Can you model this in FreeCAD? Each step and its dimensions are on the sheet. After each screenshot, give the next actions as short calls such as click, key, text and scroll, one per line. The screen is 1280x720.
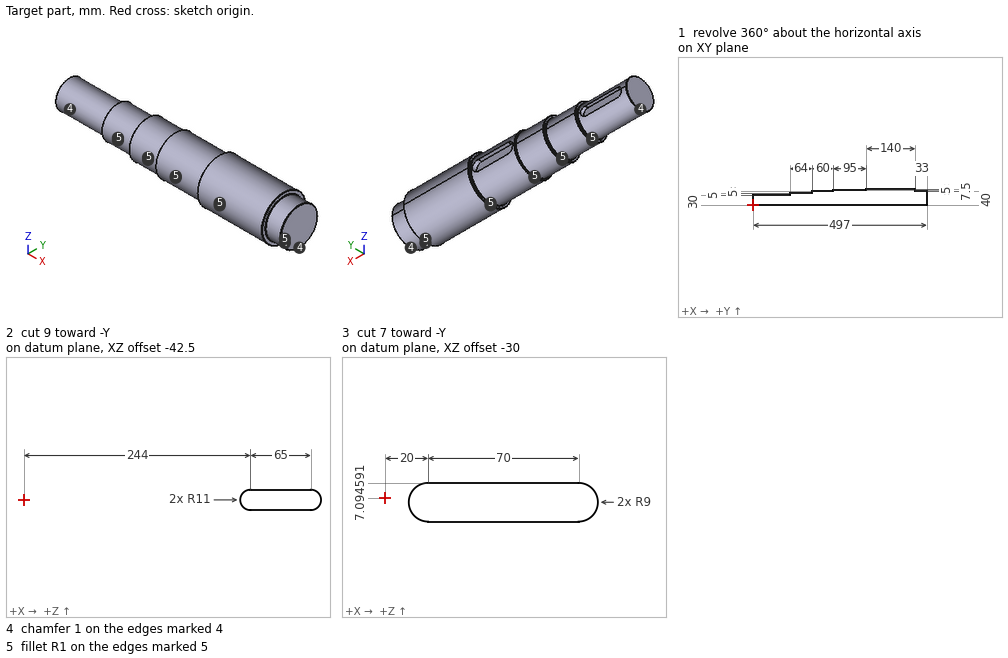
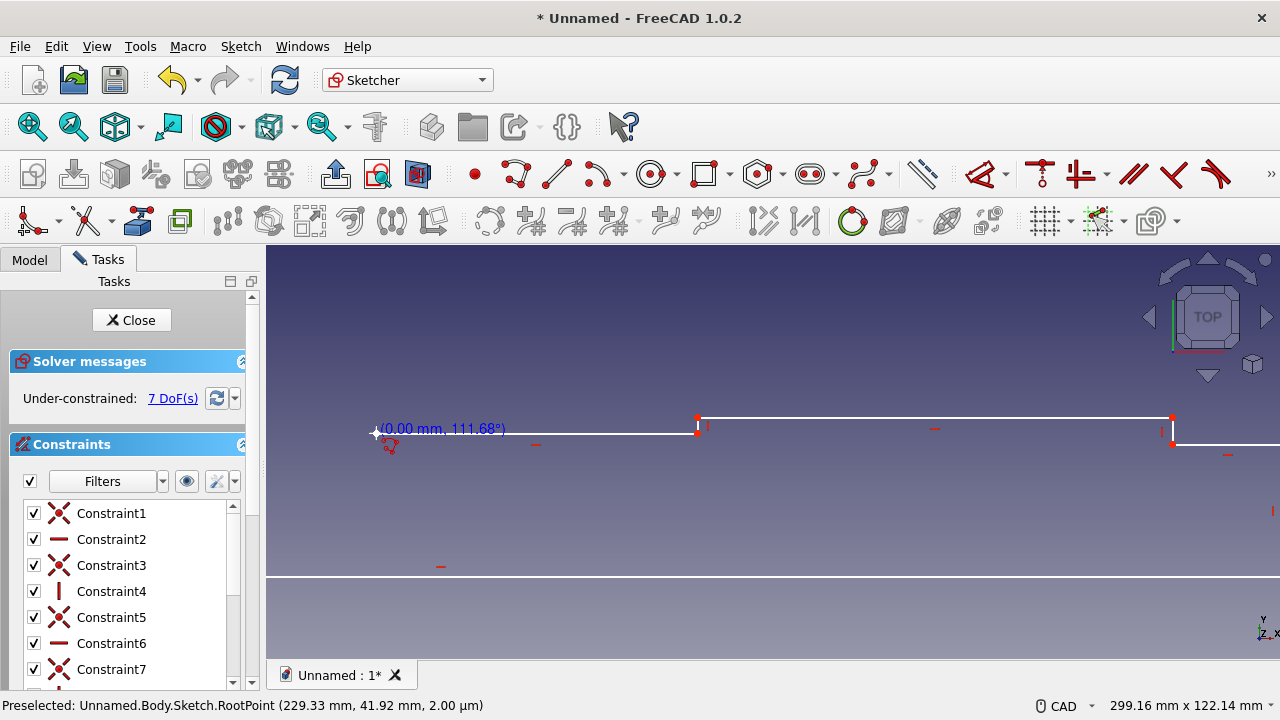
scroll(376, 442, up, 4)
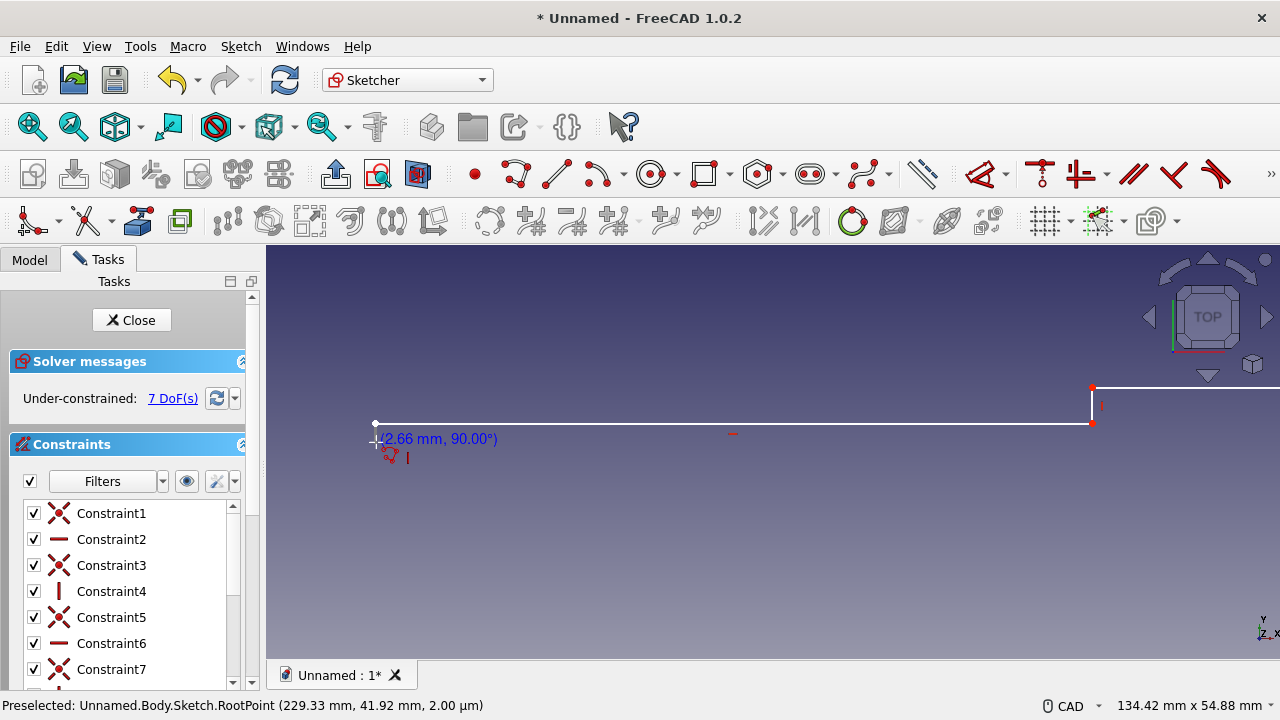
click(376, 440)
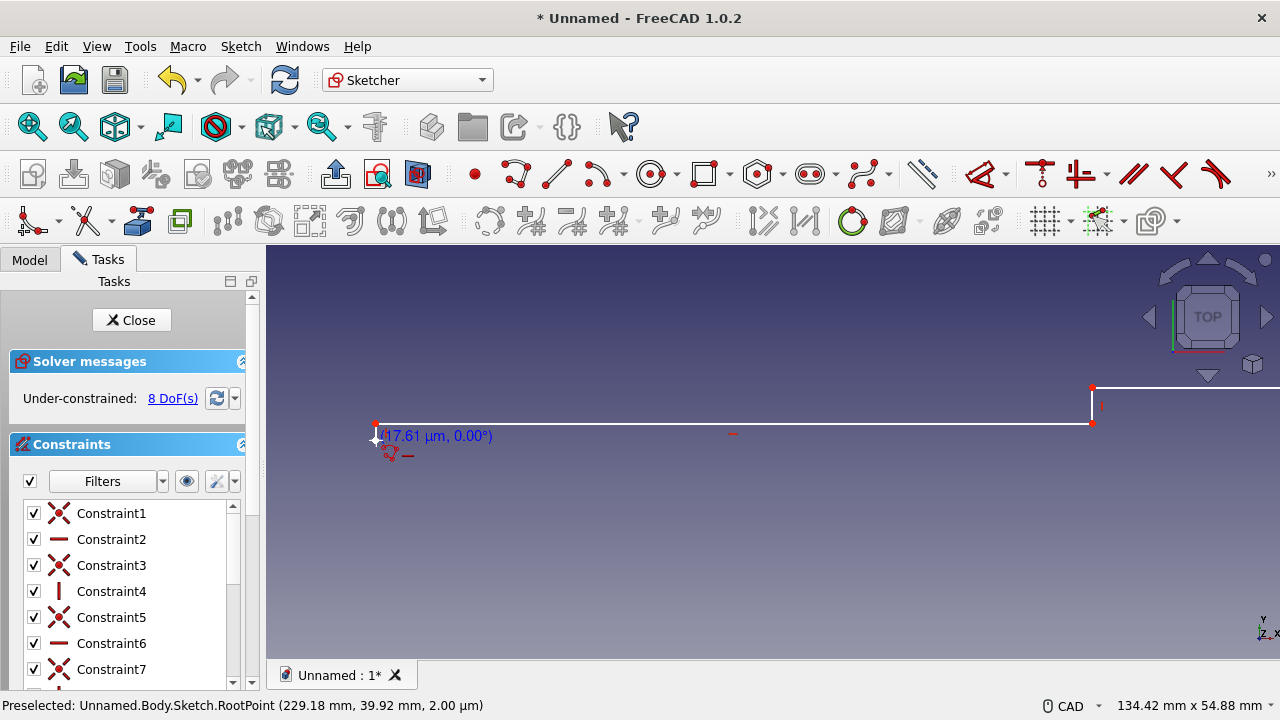
scroll(740, 430, down, 9)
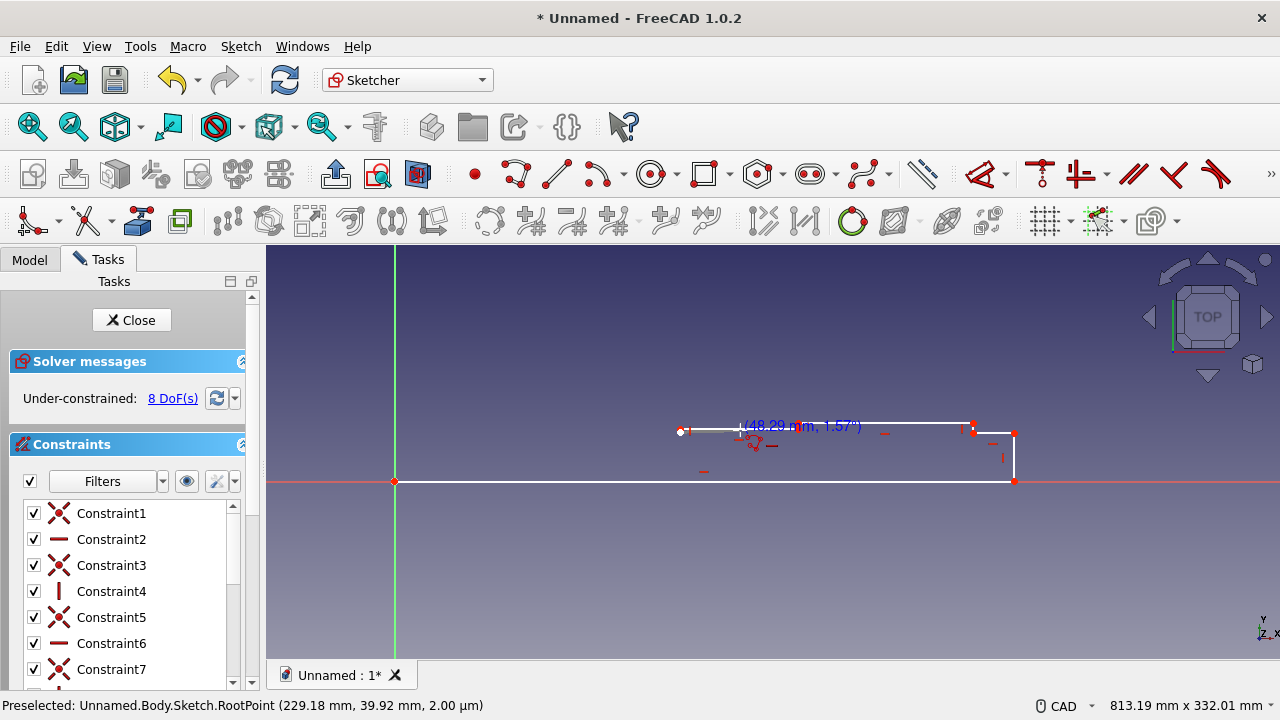
click(605, 432)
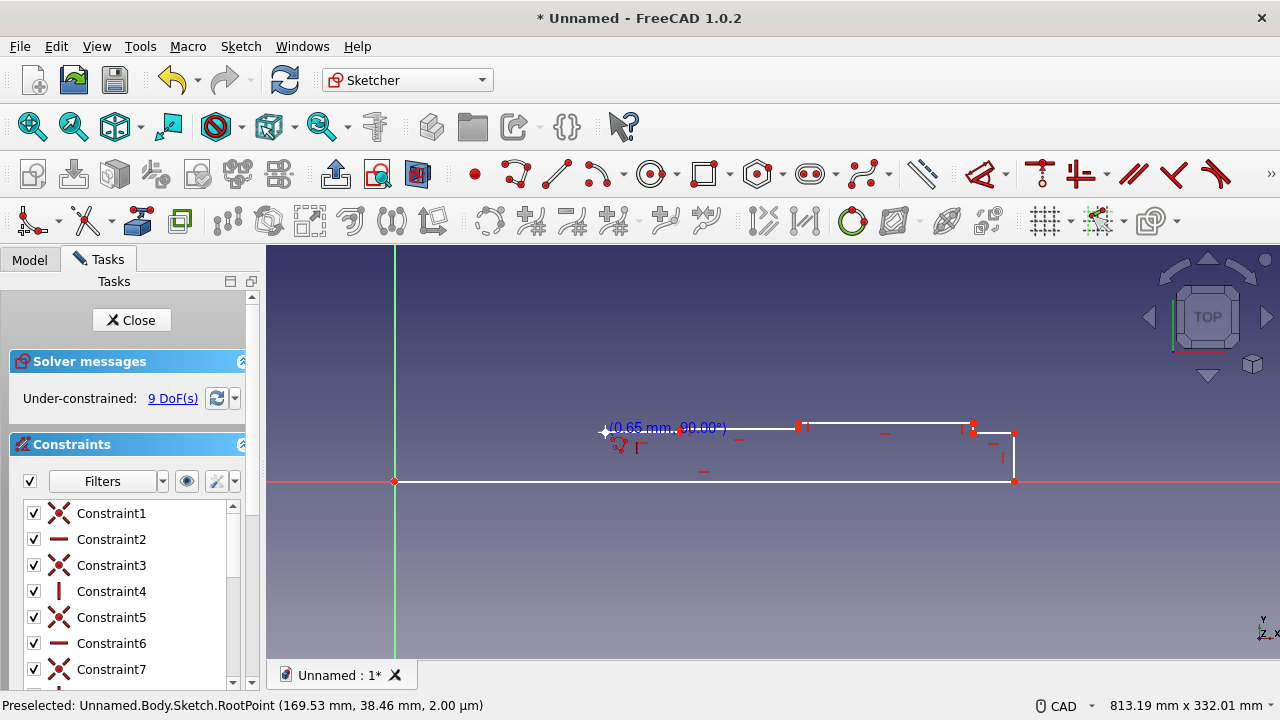
scroll(605, 438, up, 5)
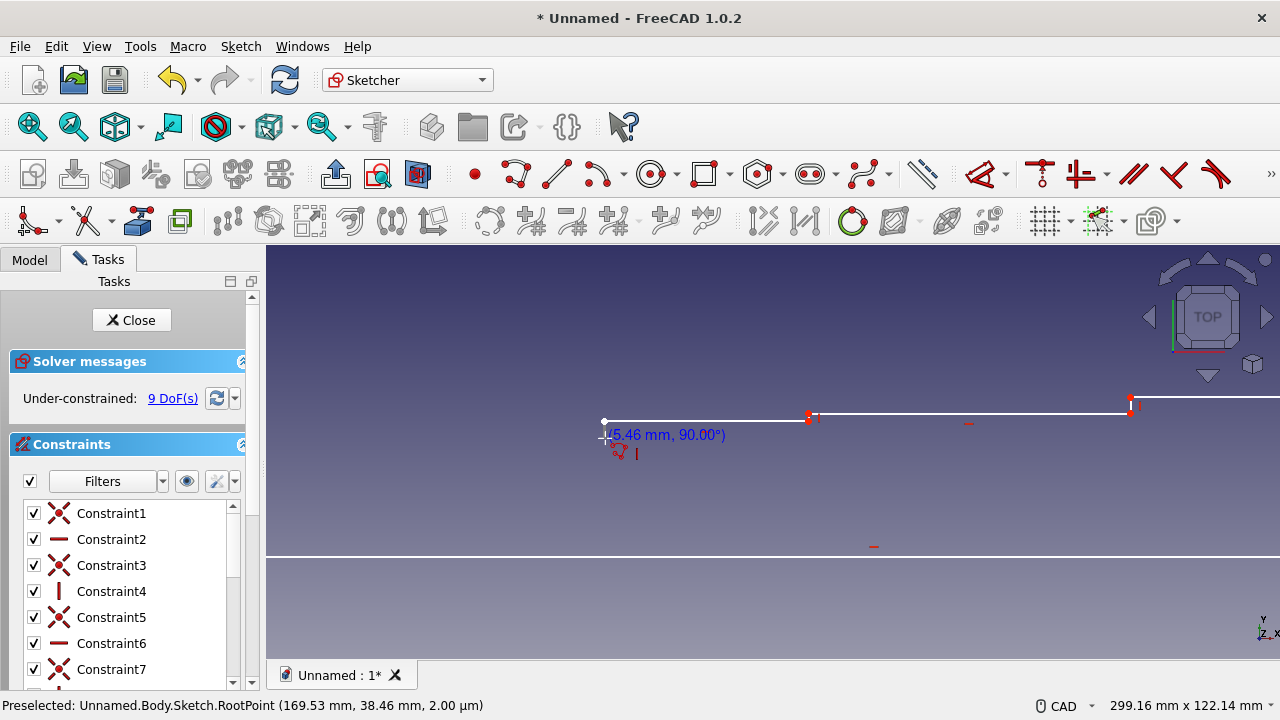
click(604, 438)
click(388, 438)
click(388, 455)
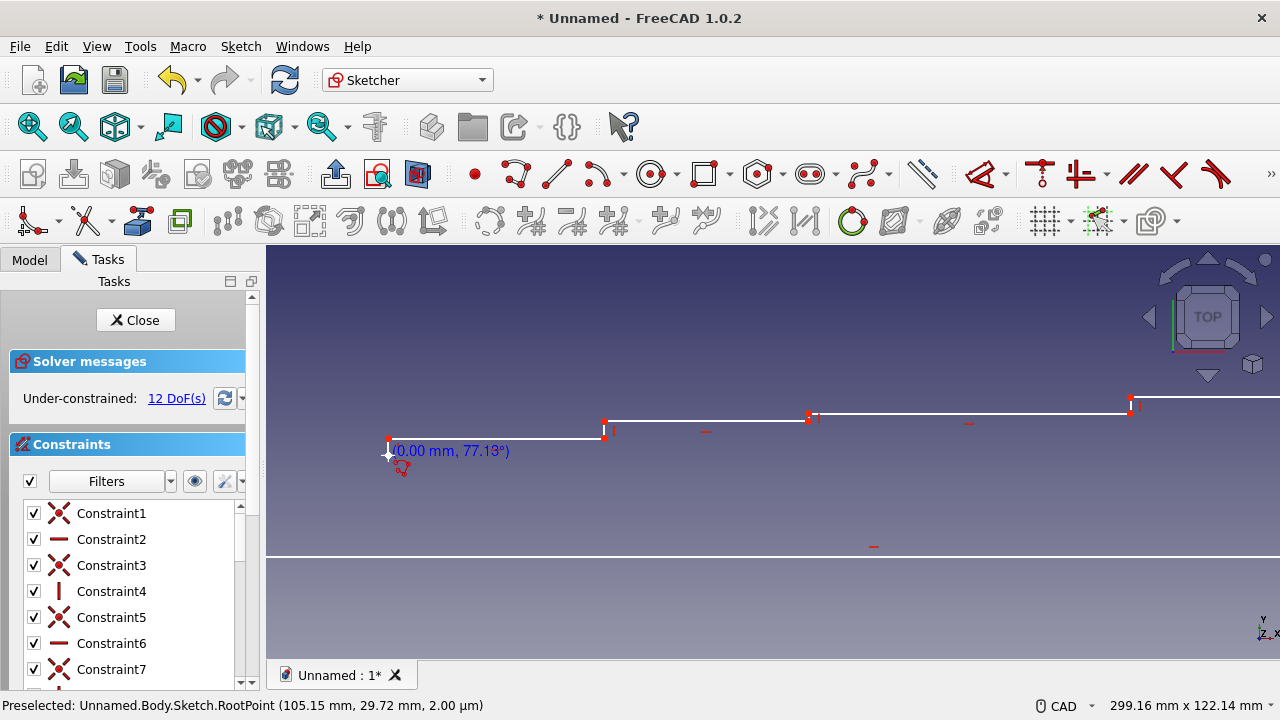
scroll(605, 438, down, 5)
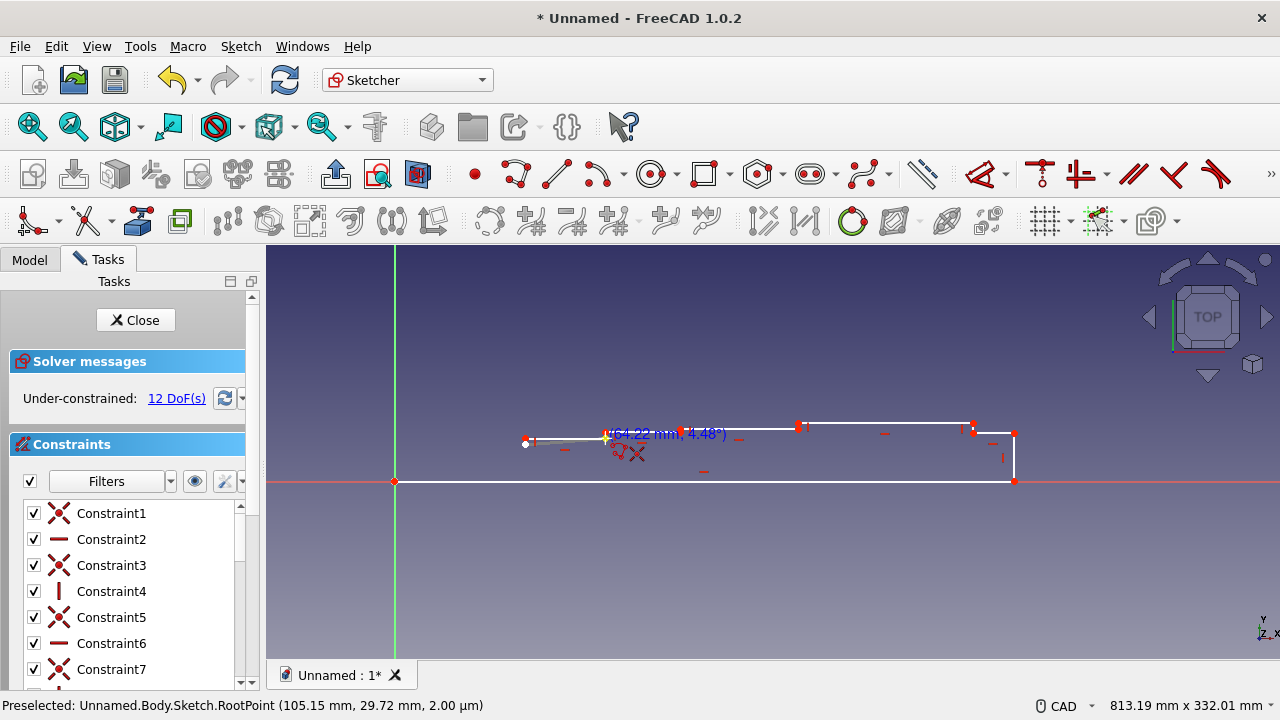
click(404, 445)
click(395, 482)
key(Escape)
key(Escape)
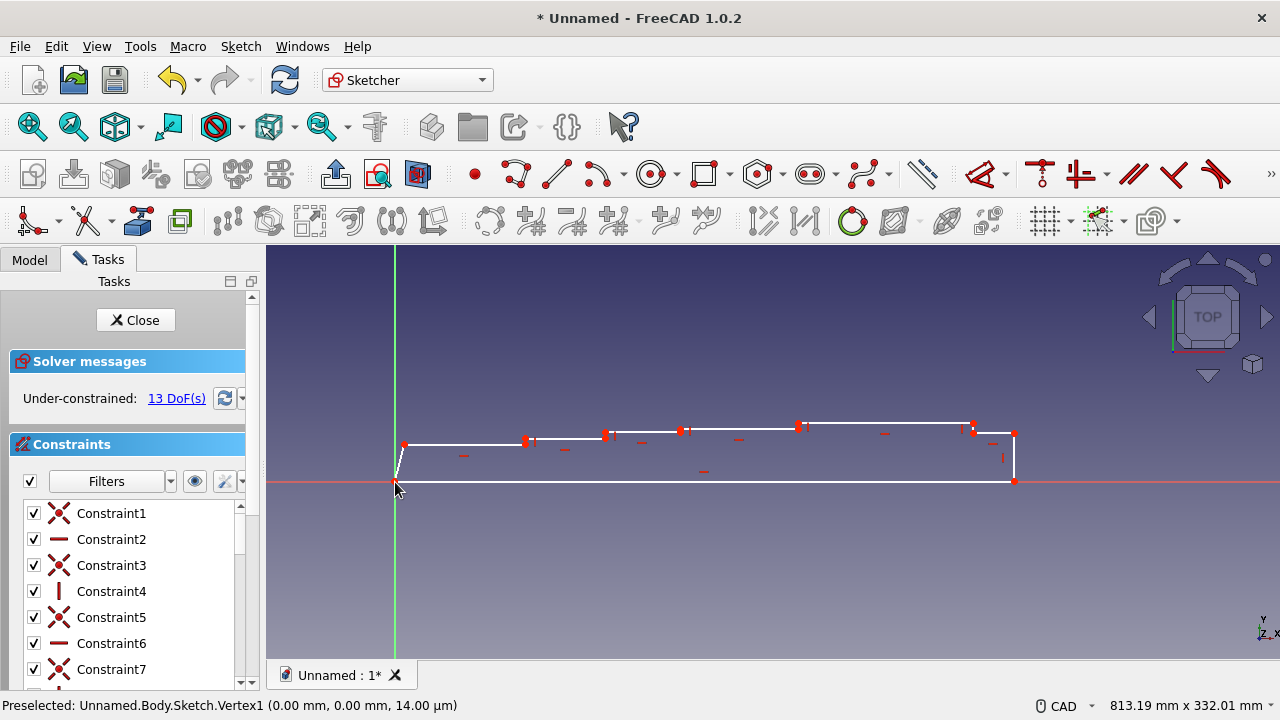
scroll(397, 471, up, 2)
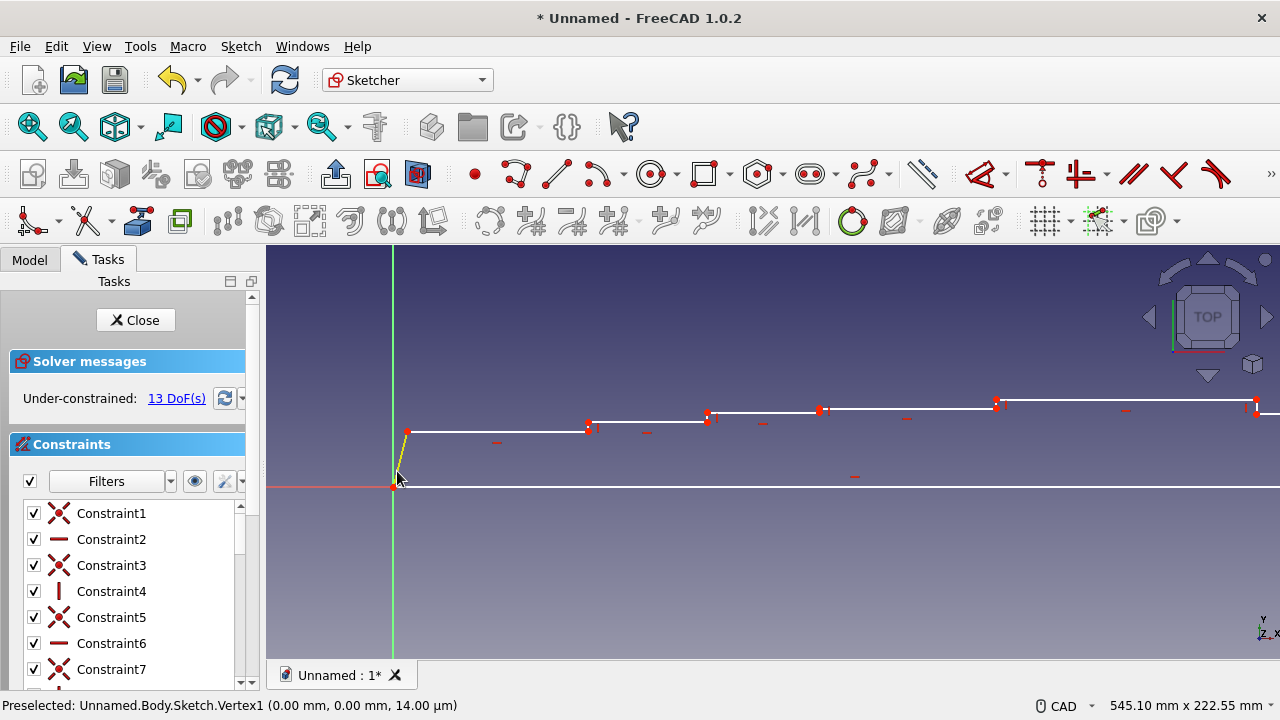
click(398, 470)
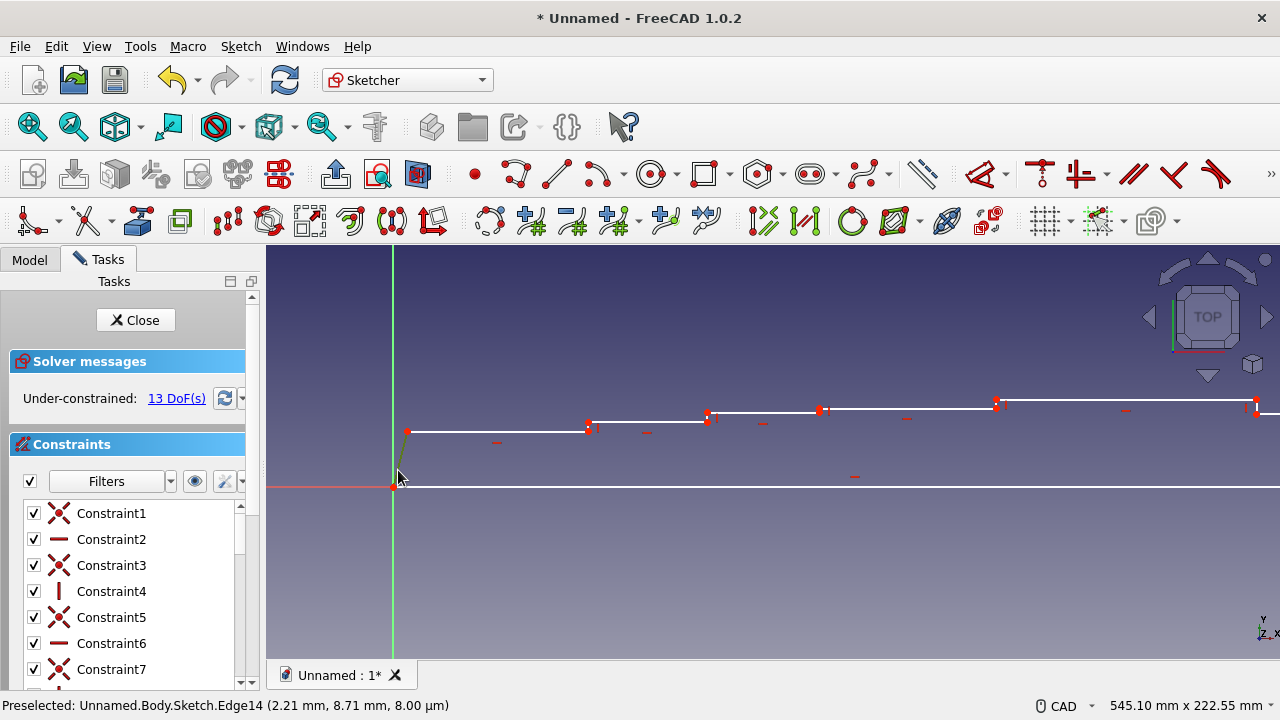
key(v)